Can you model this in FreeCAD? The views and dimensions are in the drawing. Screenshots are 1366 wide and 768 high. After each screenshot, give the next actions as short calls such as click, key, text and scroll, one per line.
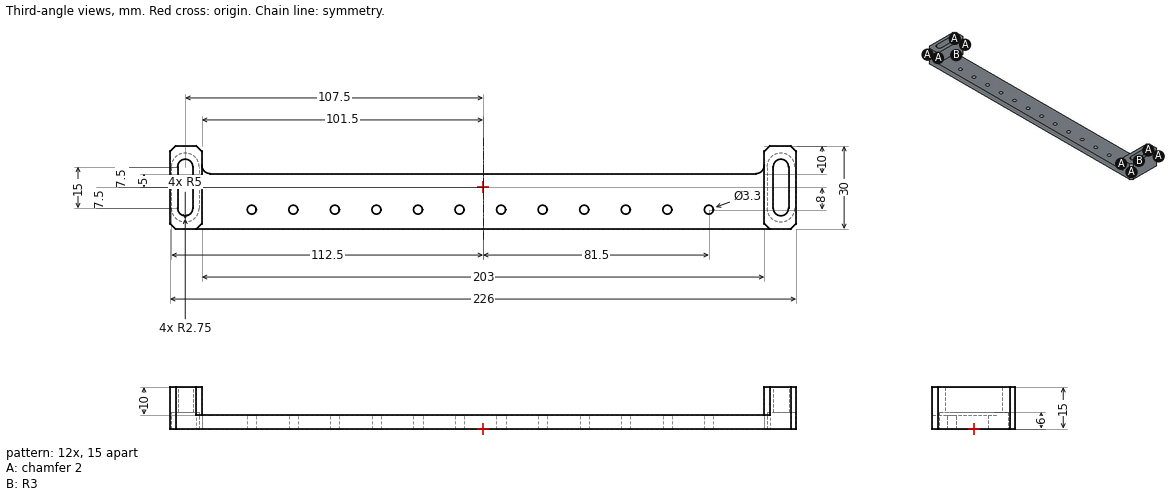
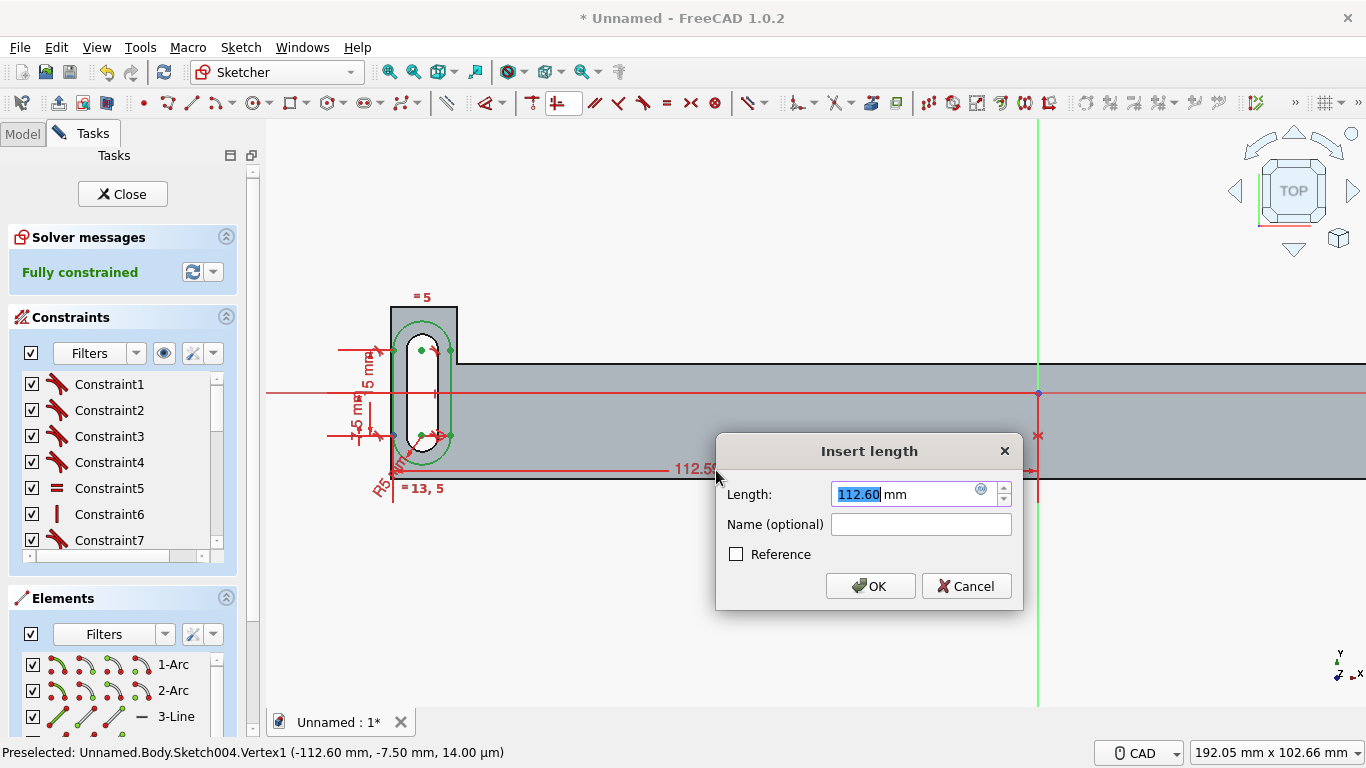
text(112.5)
key(Return)
key(Escape)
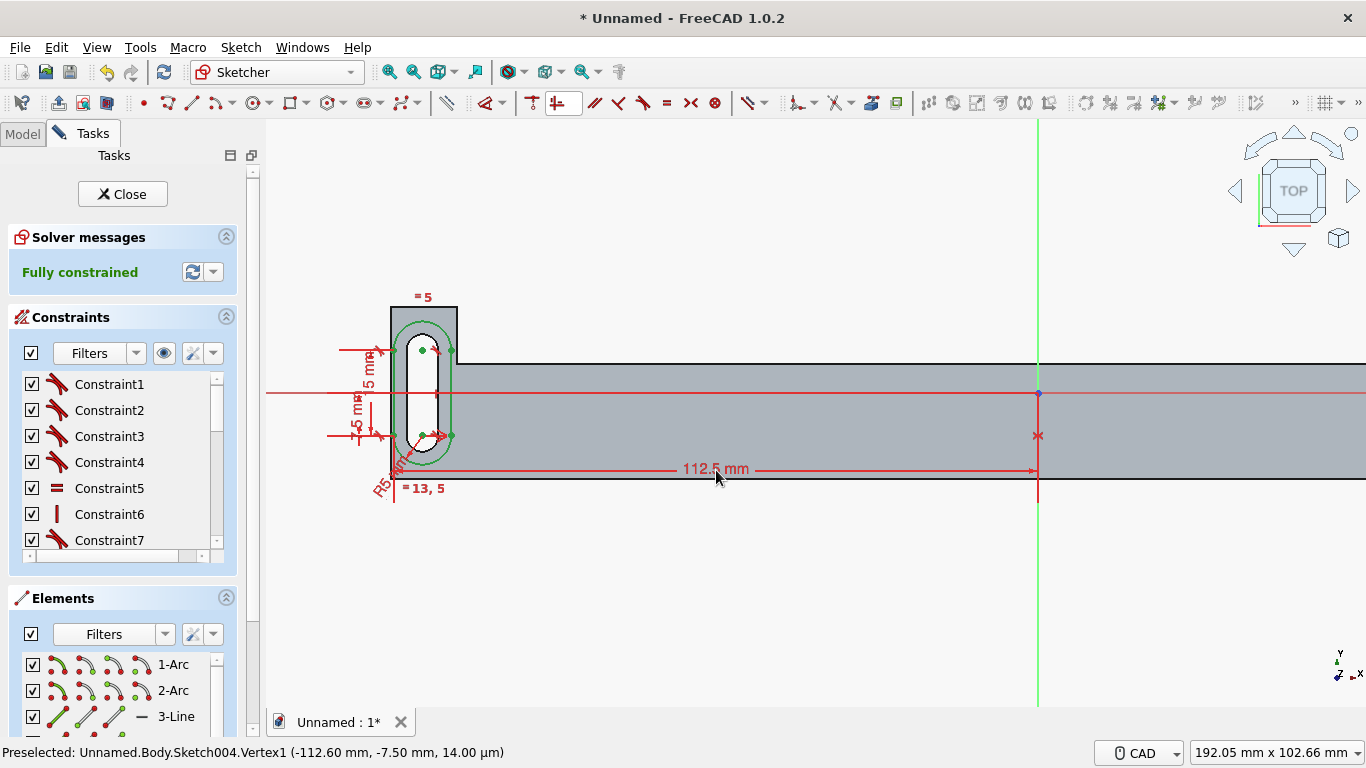
click(123, 194)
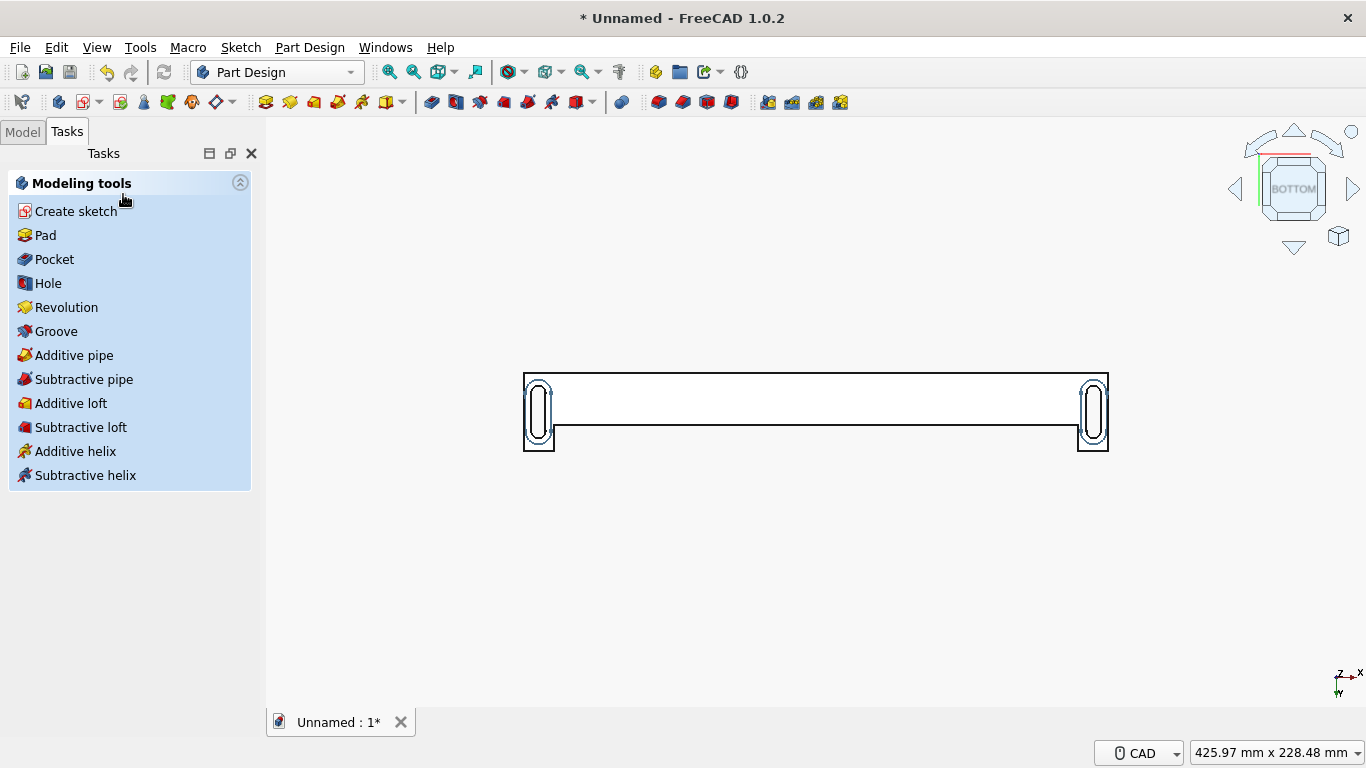
click(432, 102)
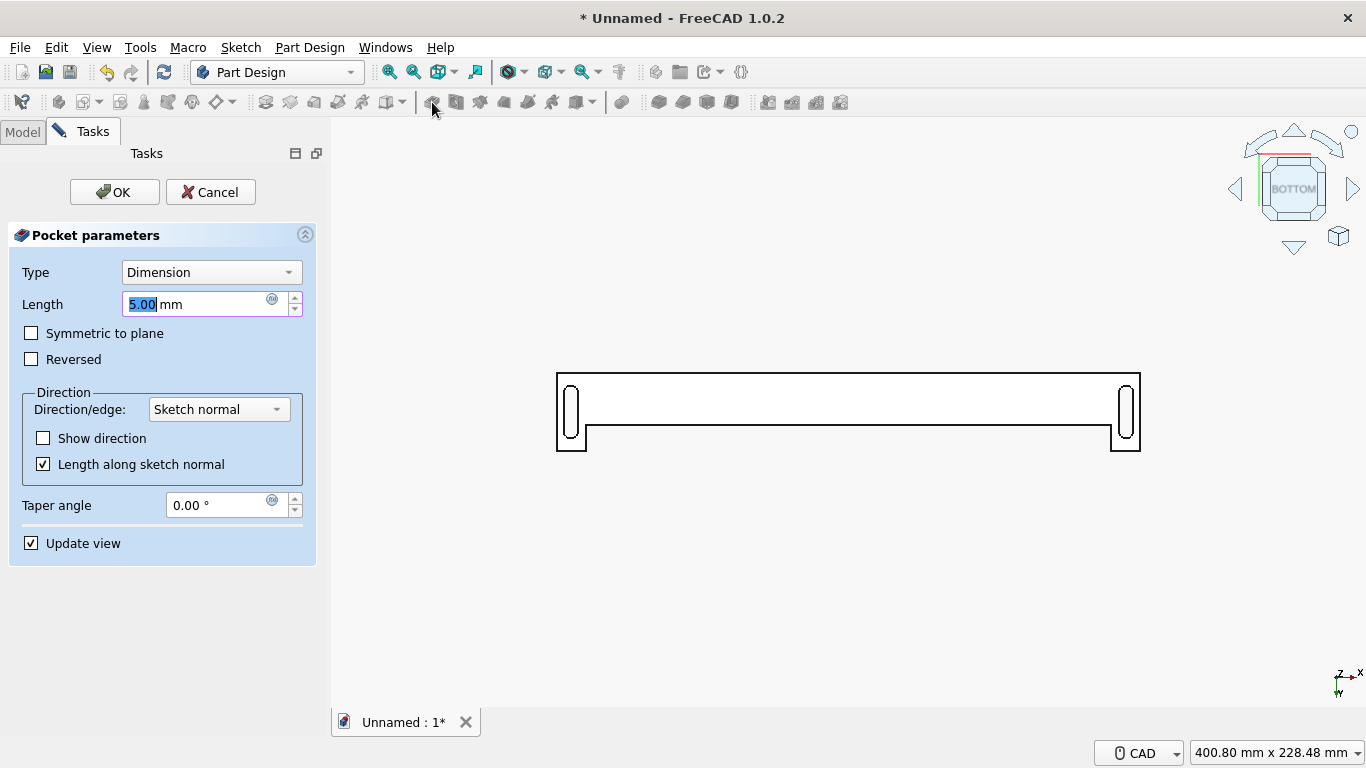
text(6)
key(Tab)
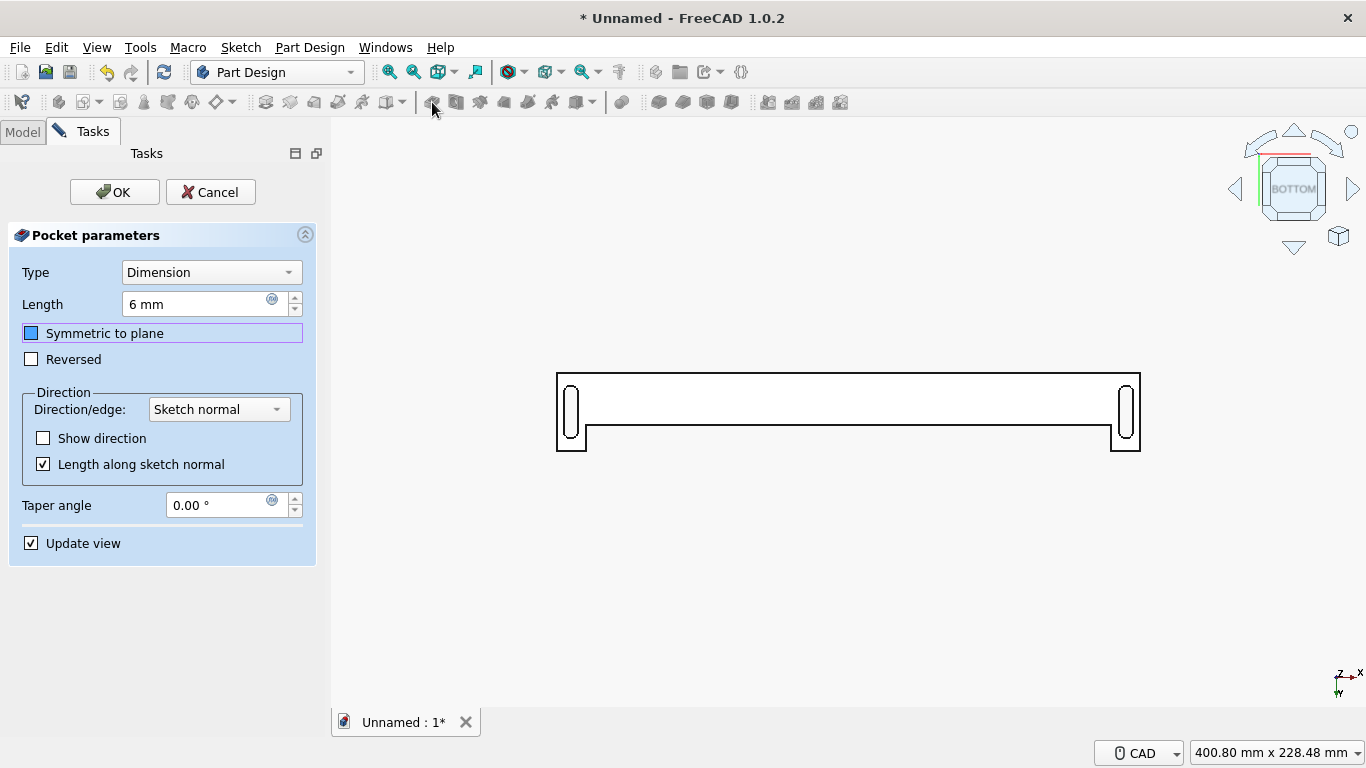
click(30, 359)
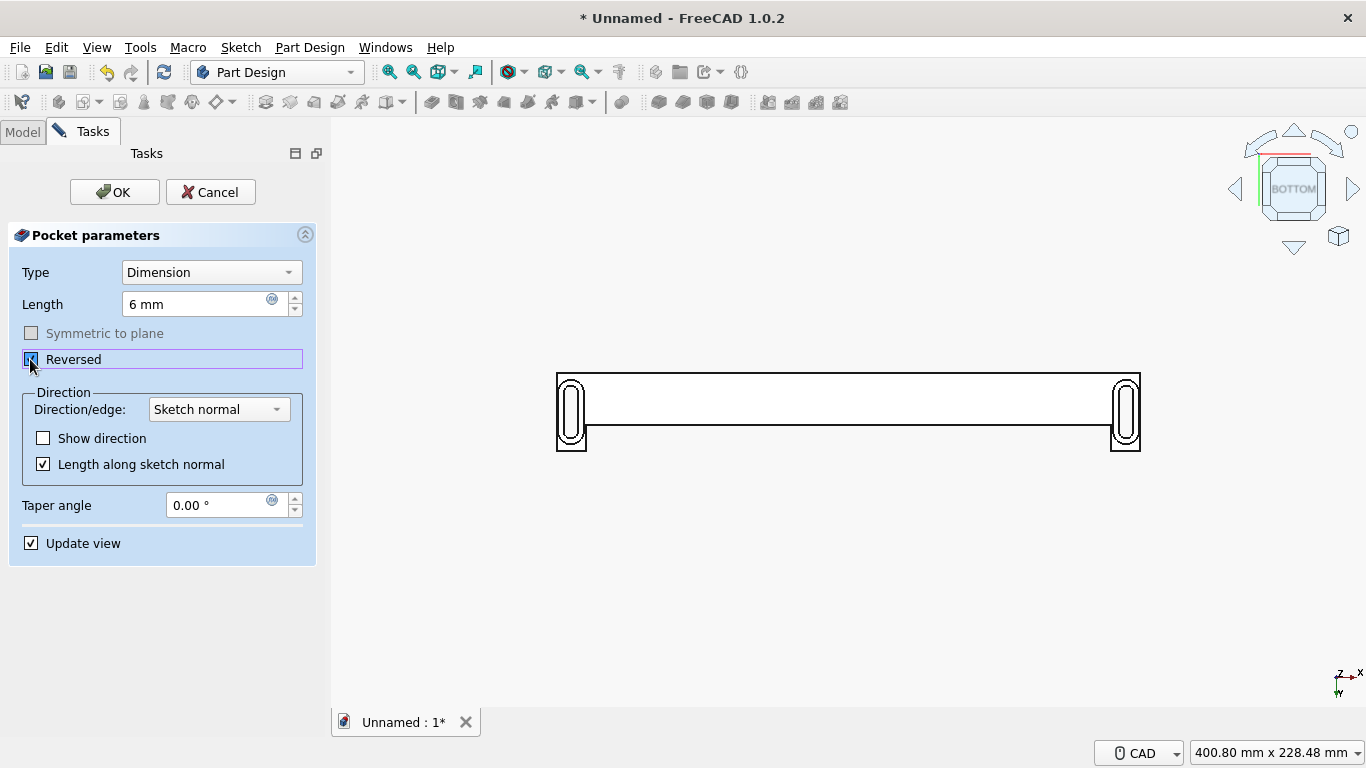
click(115, 192)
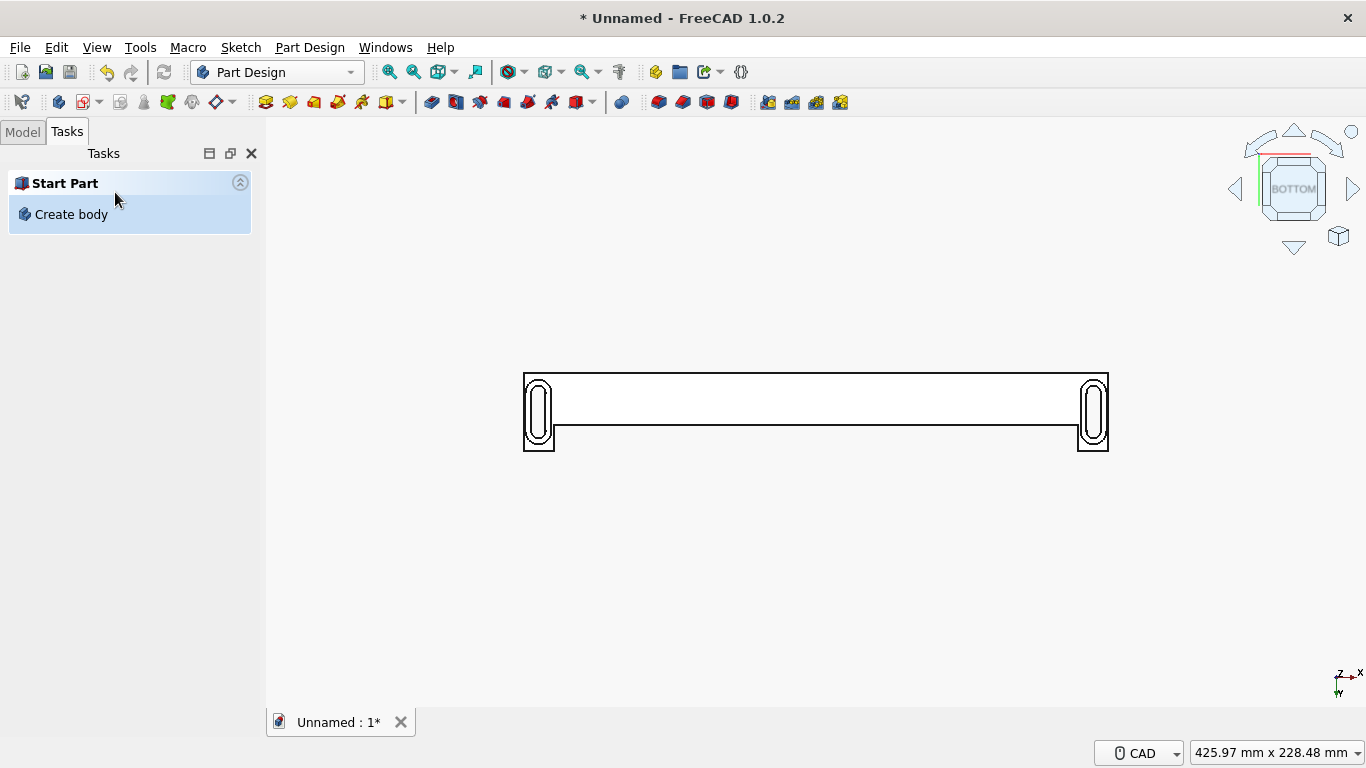
click(983, 400)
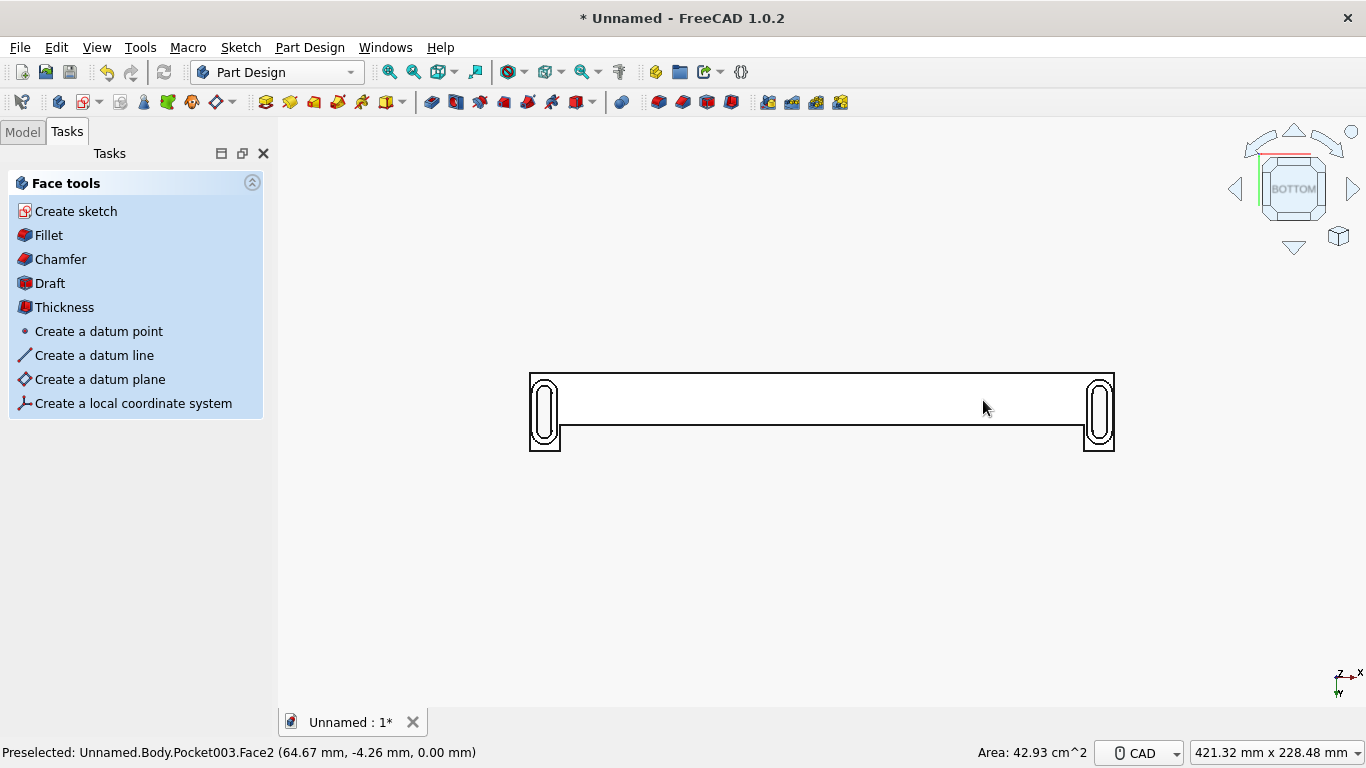
click(84, 102)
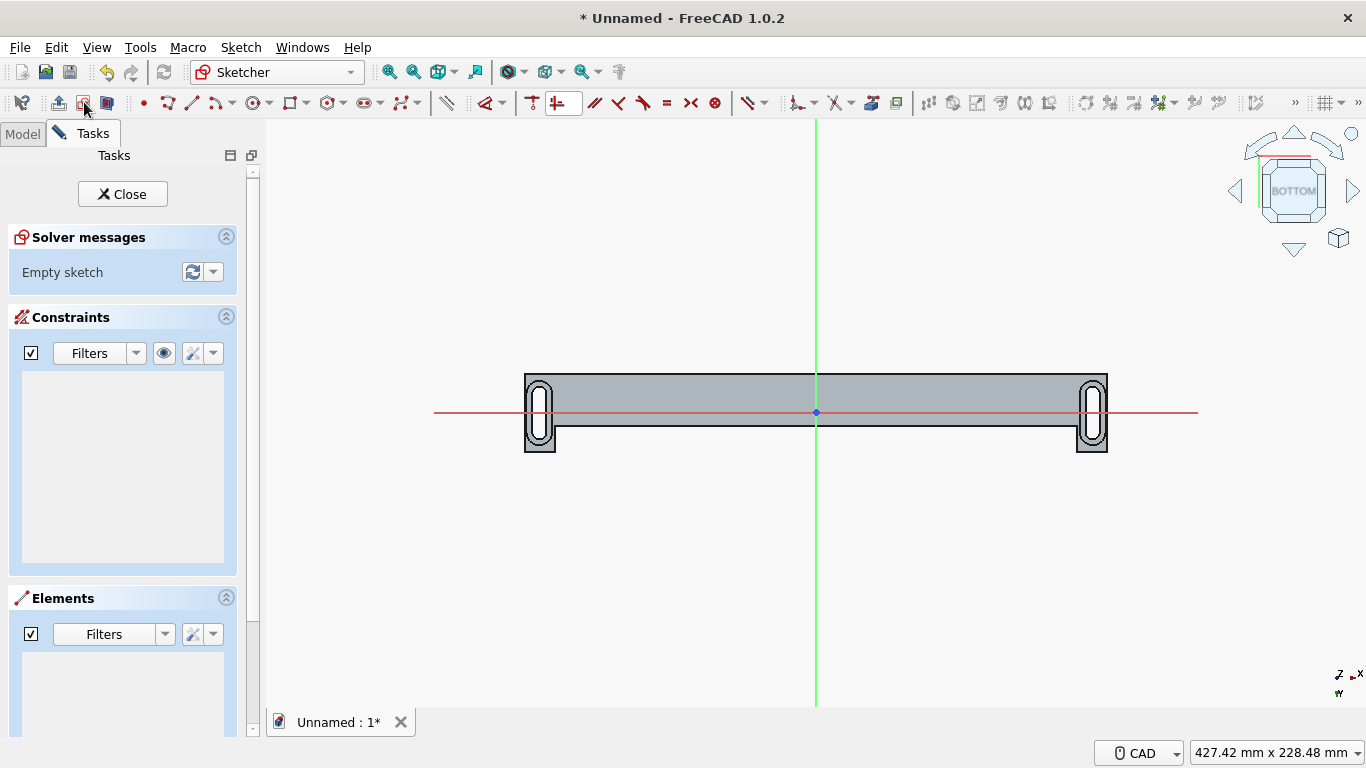
scroll(1040, 391, up, 15)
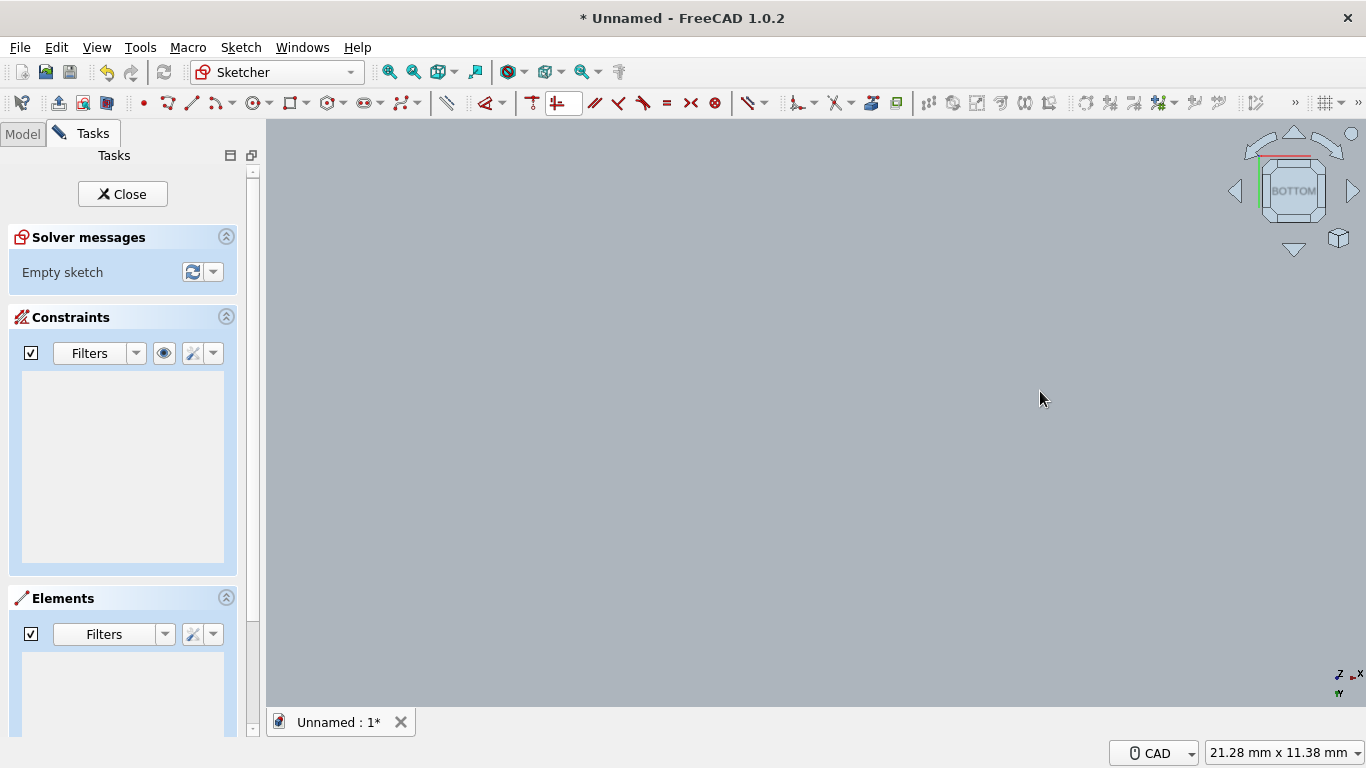
scroll(734, 408, up, 4)